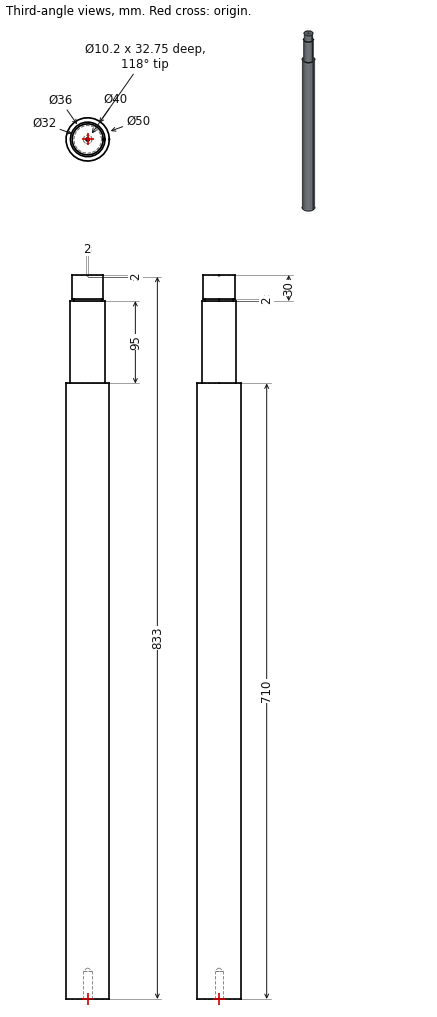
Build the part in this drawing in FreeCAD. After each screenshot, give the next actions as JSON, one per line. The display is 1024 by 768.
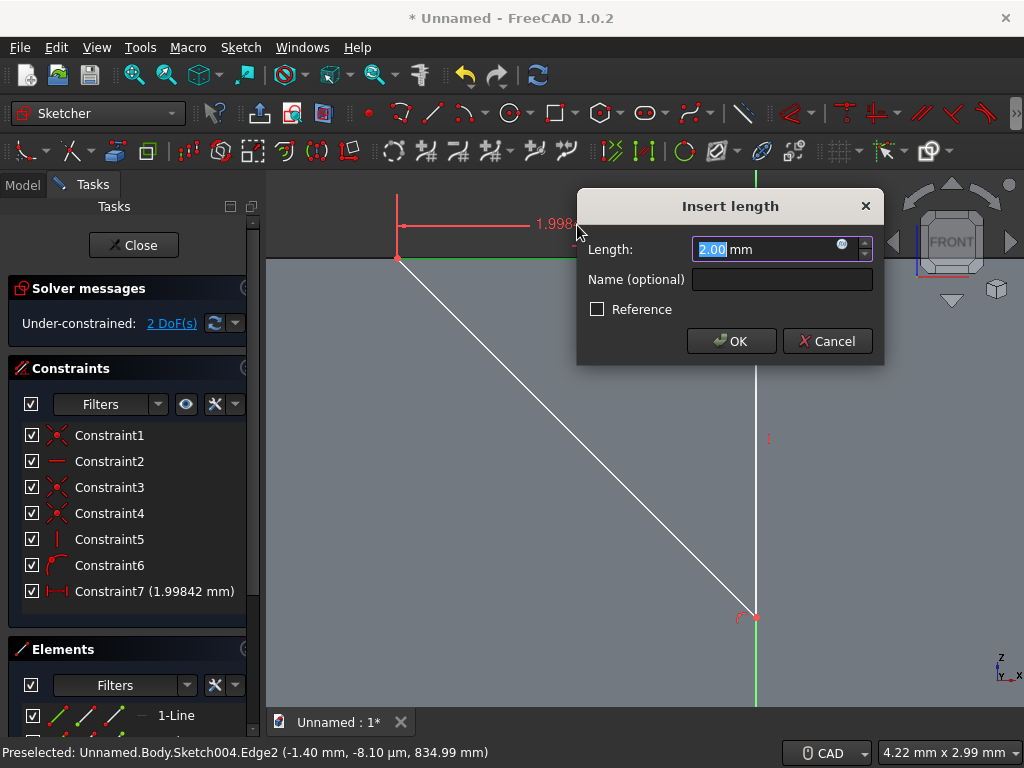
{"action": "type", "text": "2"}
{"action": "key", "text": "Return"}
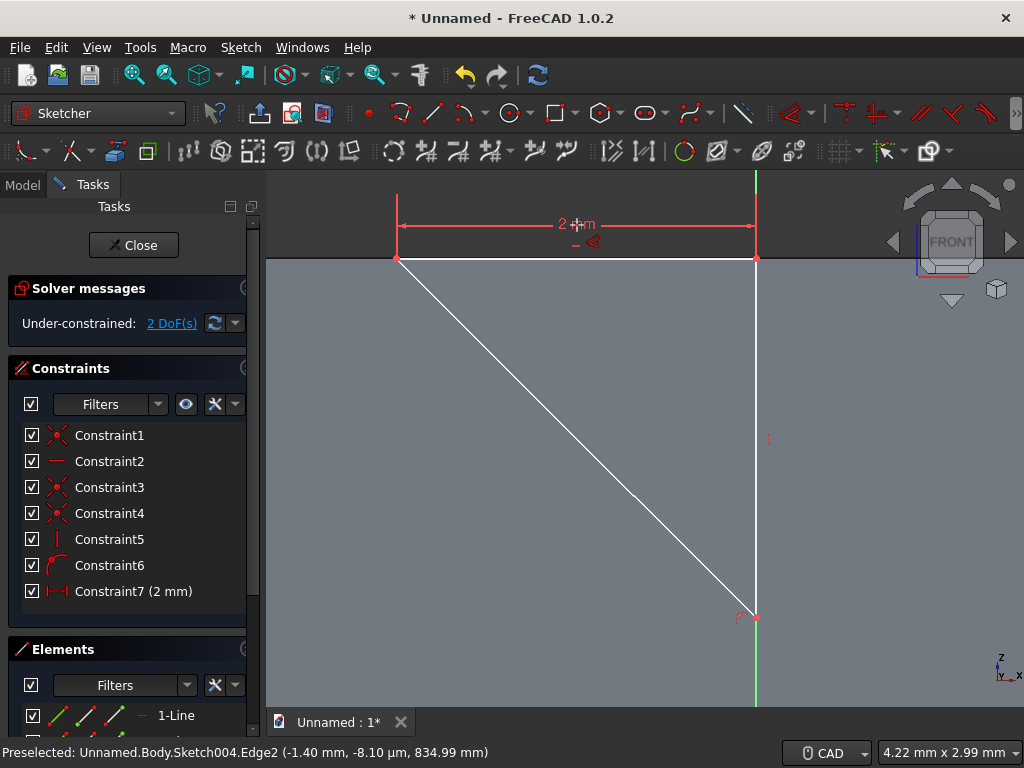
{"action": "left_click", "coordinate": [756, 367]}
{"action": "left_click", "coordinate": [790, 439]}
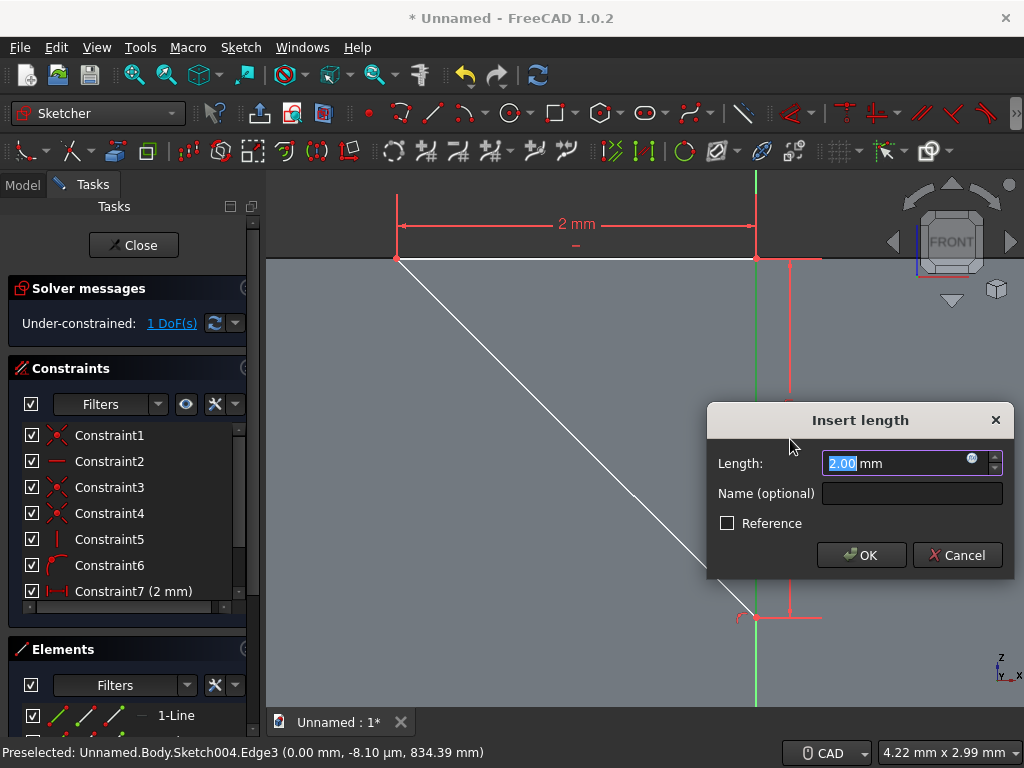
{"action": "type", "text": "2"}
{"action": "key", "text": "Return"}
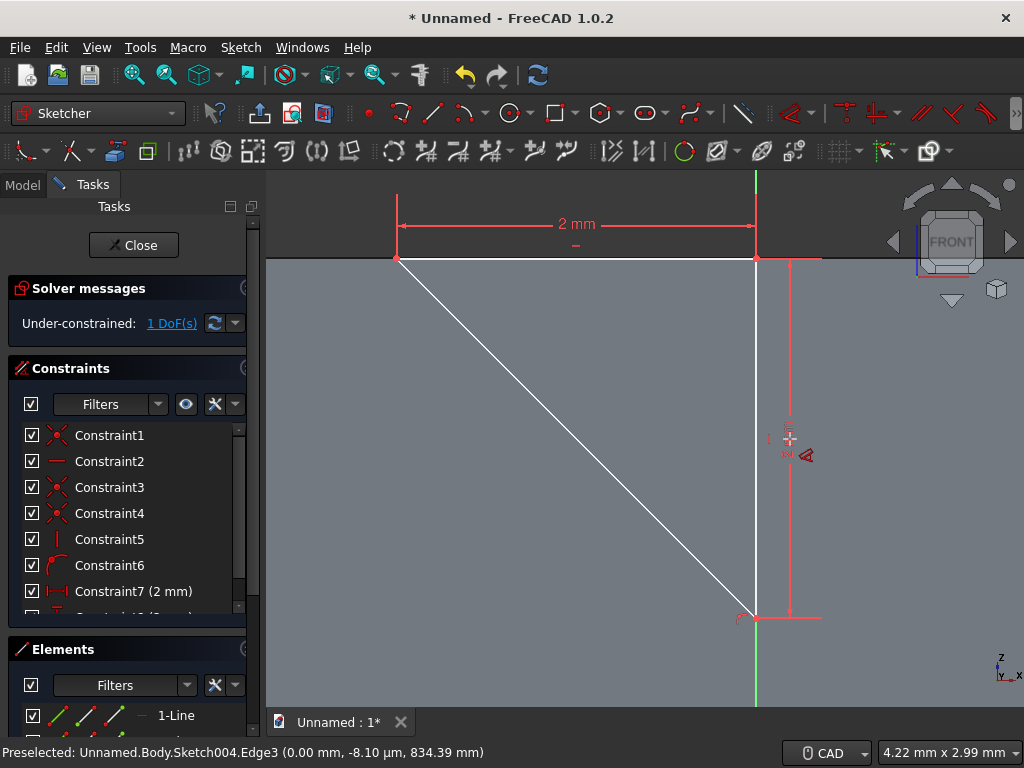
{"action": "left_click", "coordinate": [756, 618]}
{"action": "left_click", "coordinate": [790, 649]}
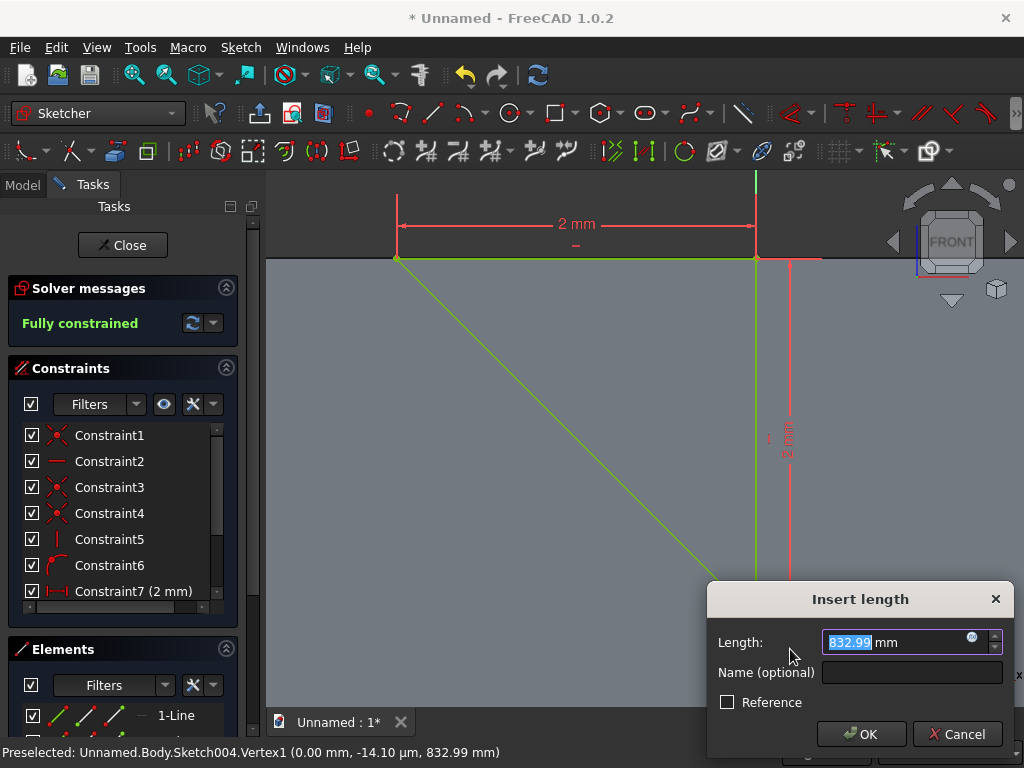
{"action": "type", "text": "833"}
{"action": "key", "text": "Return"}
{"action": "key", "text": "Escape"}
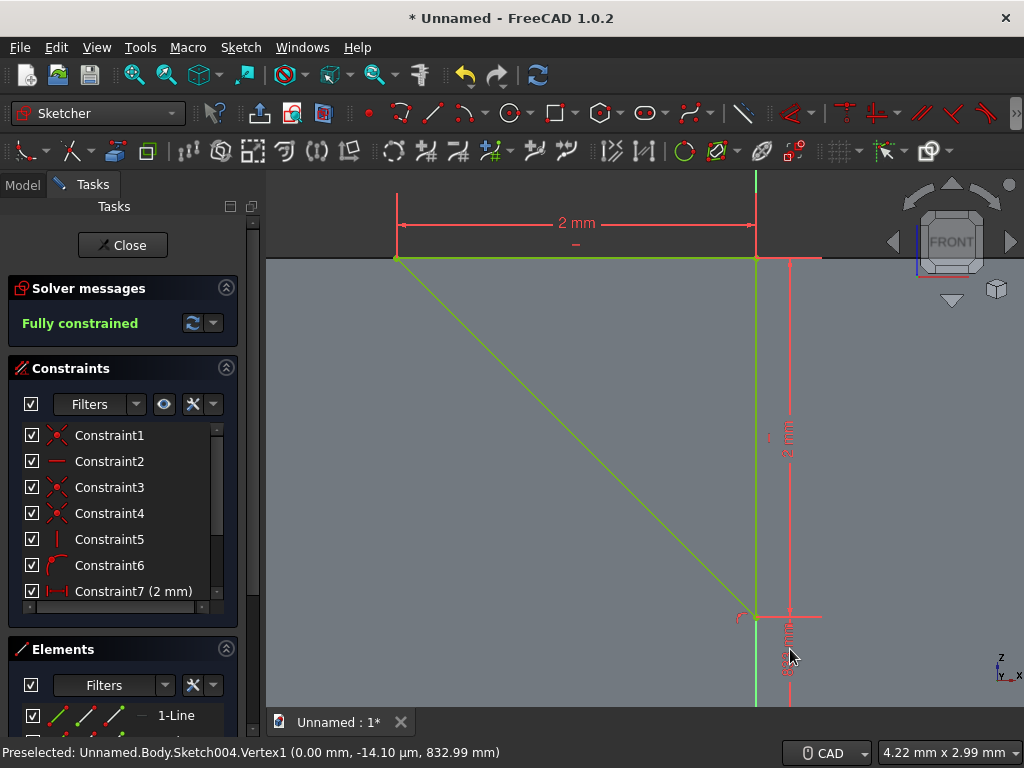
{"action": "left_click", "coordinate": [123, 245]}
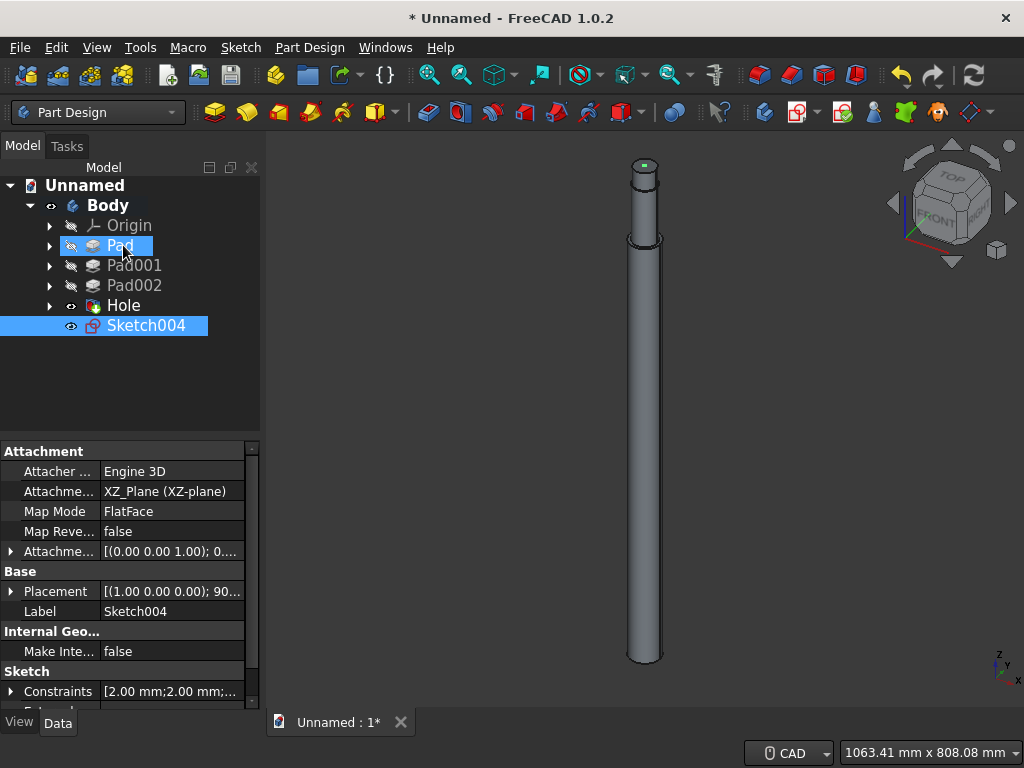
{"action": "left_click", "coordinate": [494, 112]}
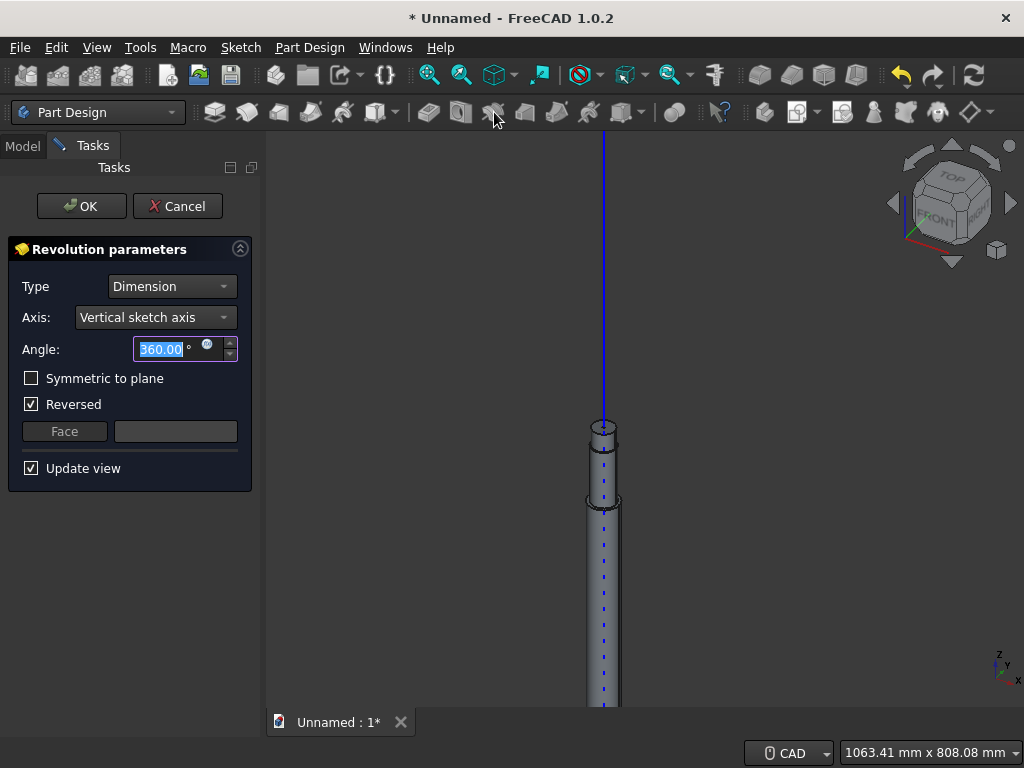
{"action": "left_click", "coordinate": [82, 206]}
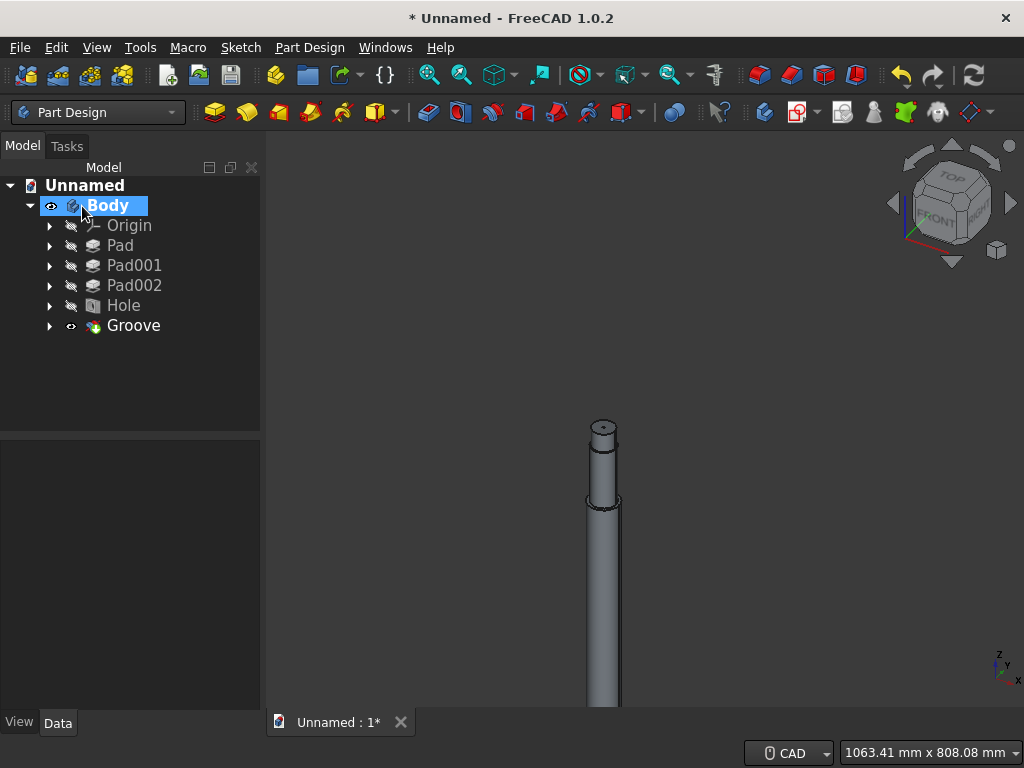
{"action": "left_click", "coordinate": [430, 76]}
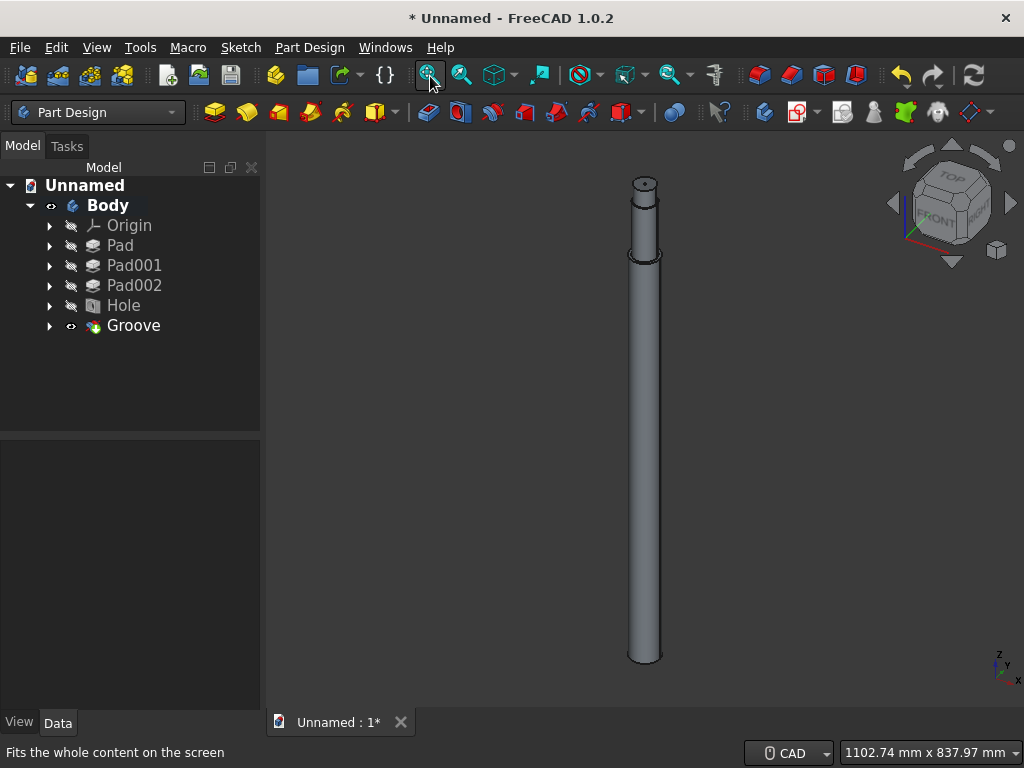
{"action": "scroll", "coordinate": [657, 201], "scroll_direction": "up", "scroll_amount": 15}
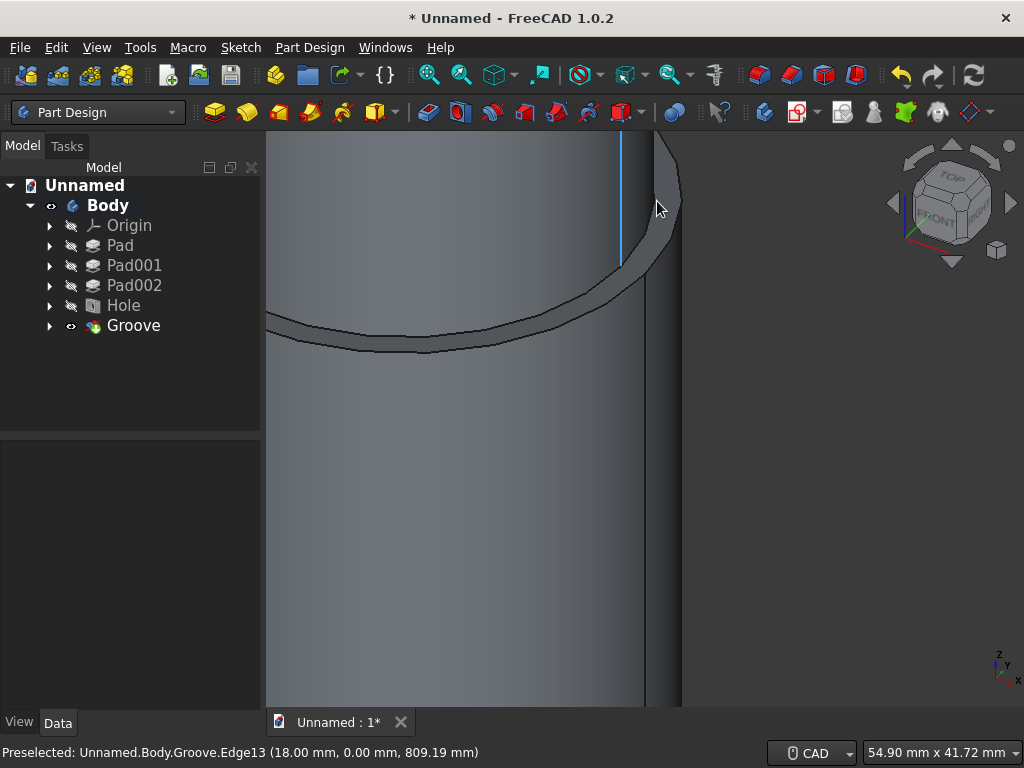
{"action": "scroll", "coordinate": [651, 223], "scroll_direction": "up", "scroll_amount": 13}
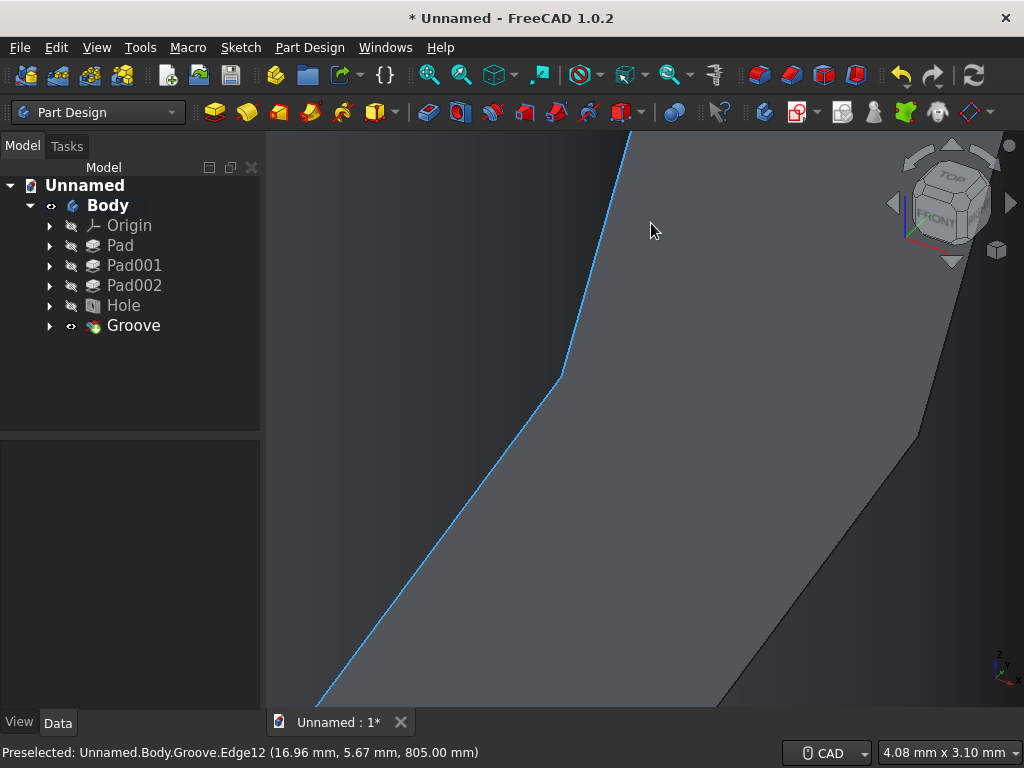
{"action": "left_click", "coordinate": [638, 228]}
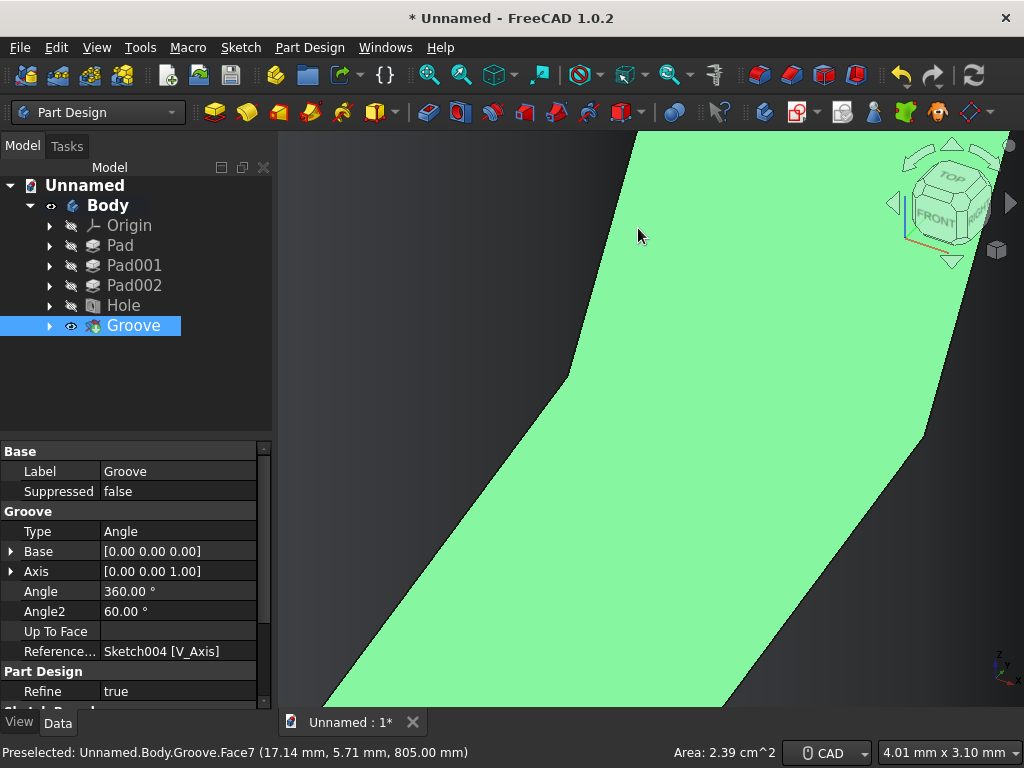
{"action": "left_click", "coordinate": [798, 112]}